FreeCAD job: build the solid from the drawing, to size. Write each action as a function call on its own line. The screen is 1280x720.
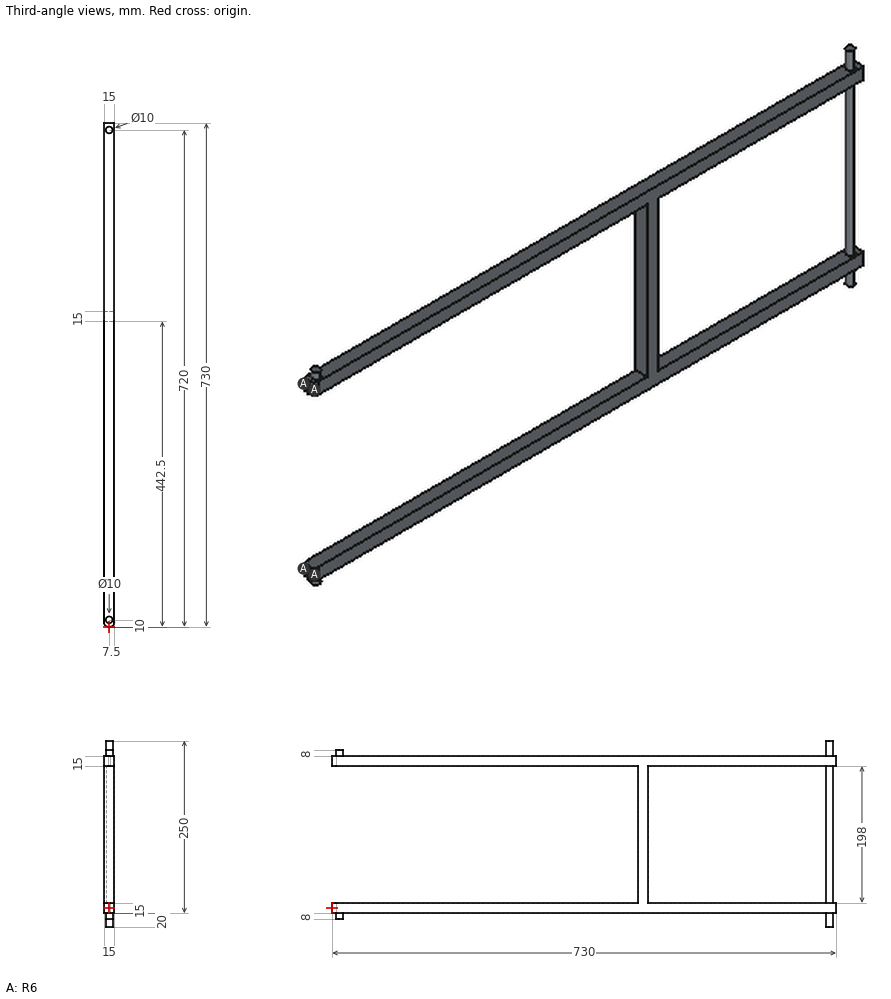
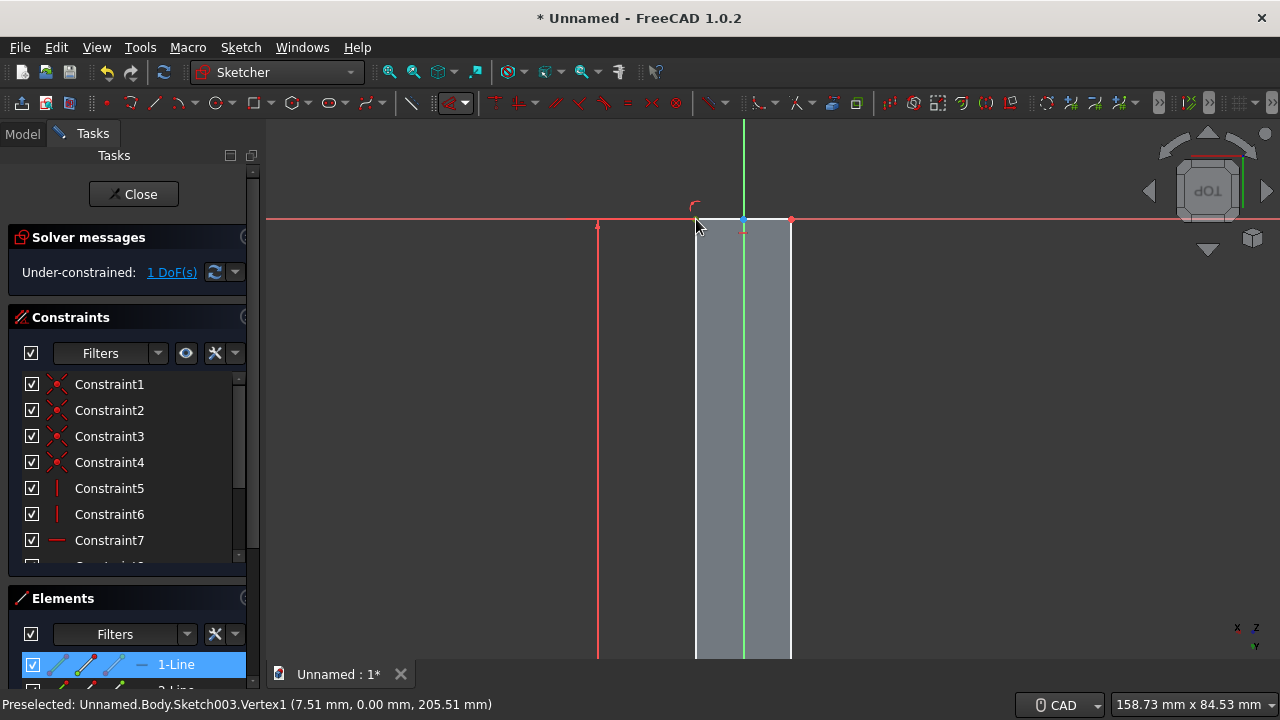
key(l)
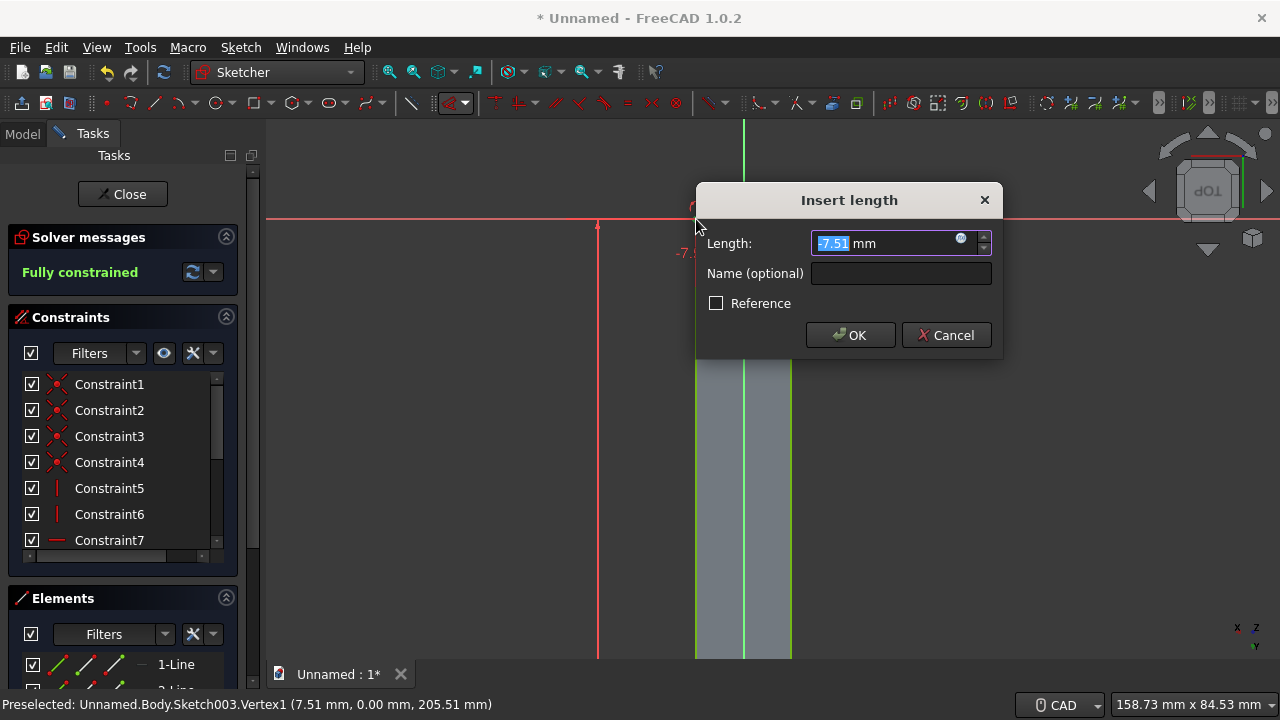
text(-7.5)
key(Return)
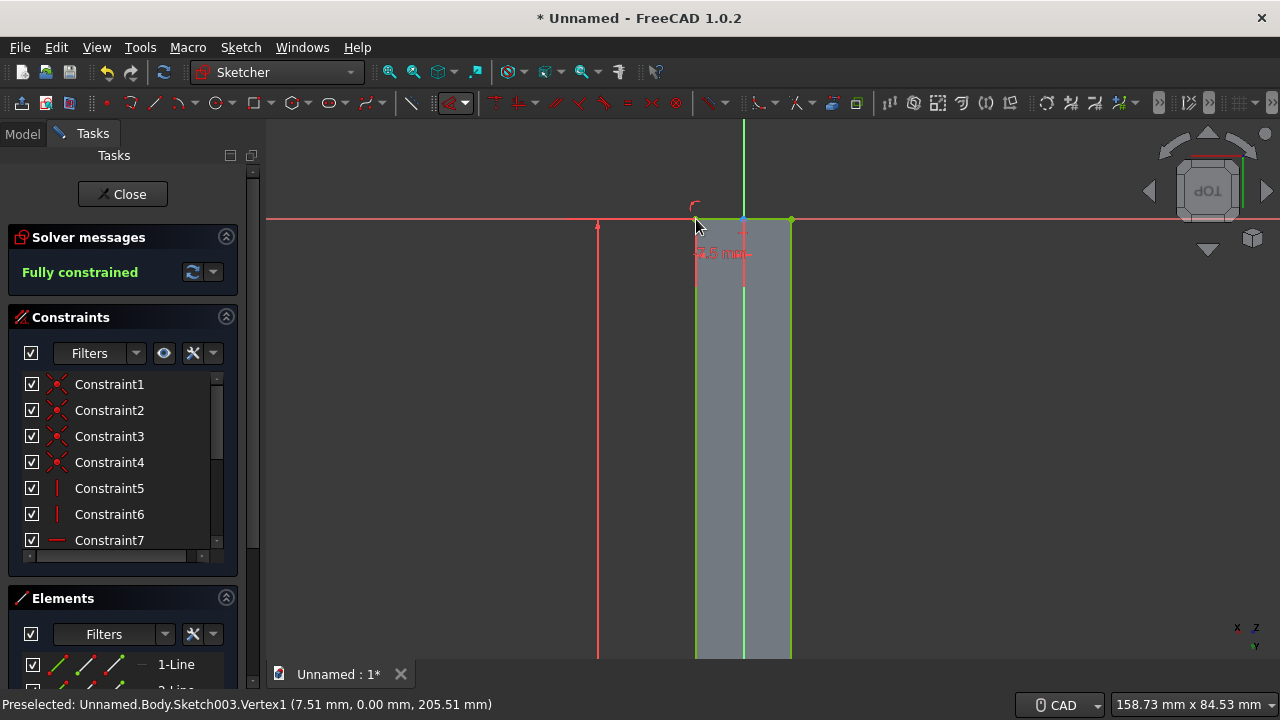
click(123, 194)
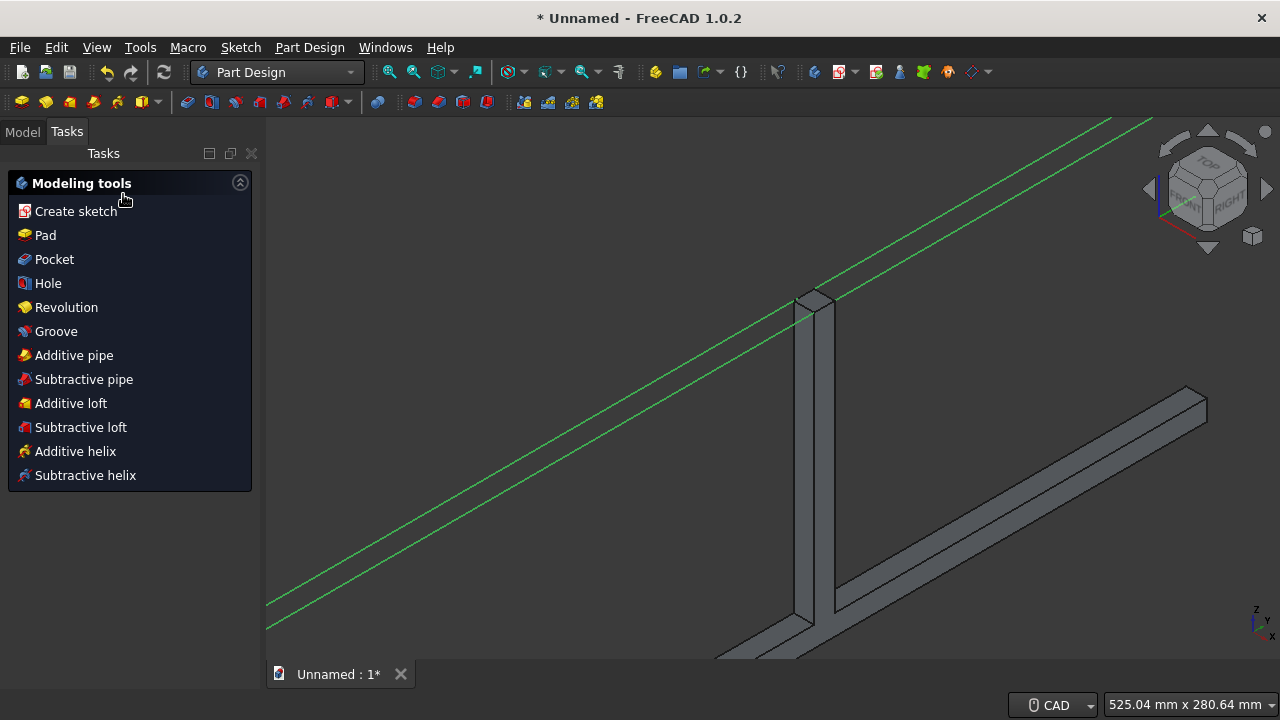
click(22, 102)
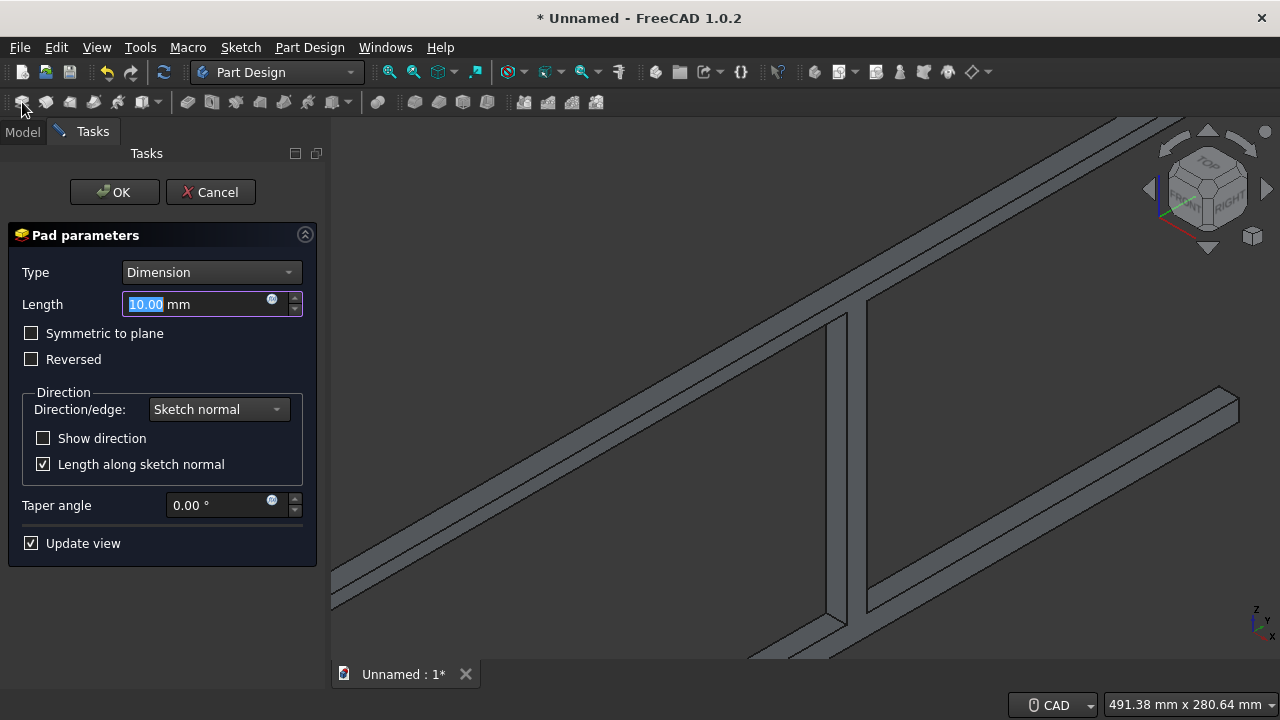
text(15)
key(Tab)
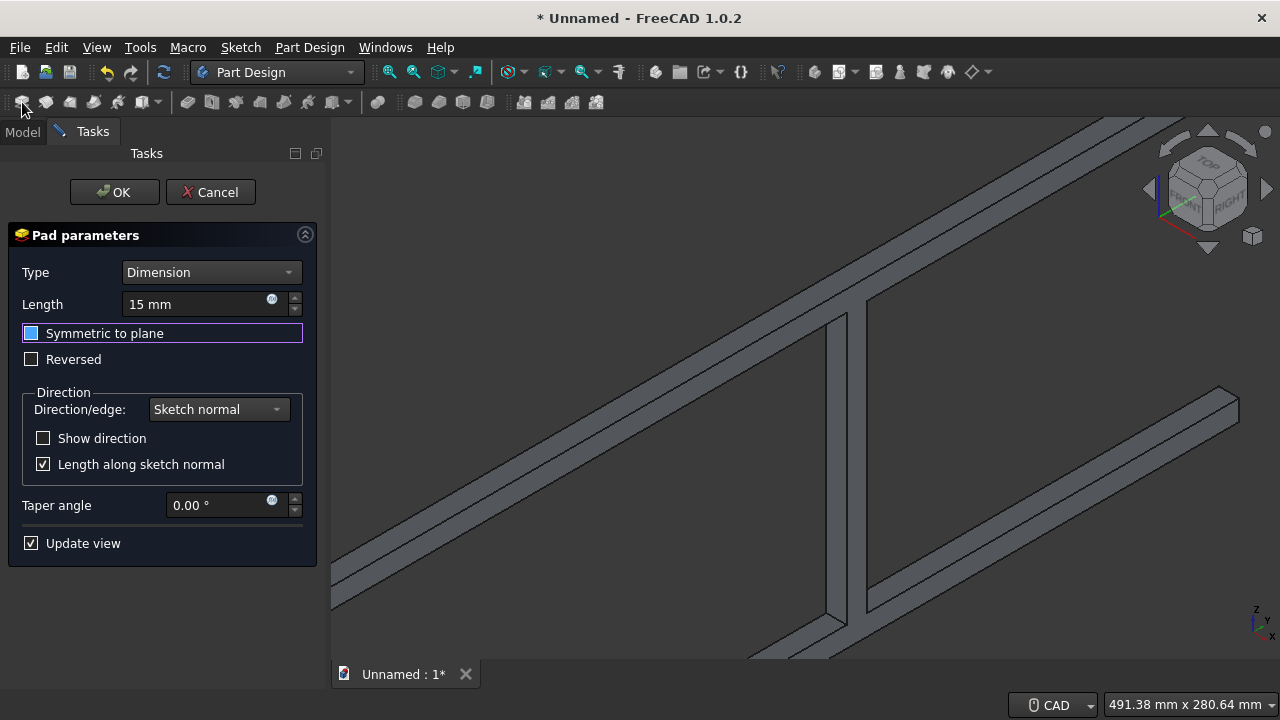
click(115, 192)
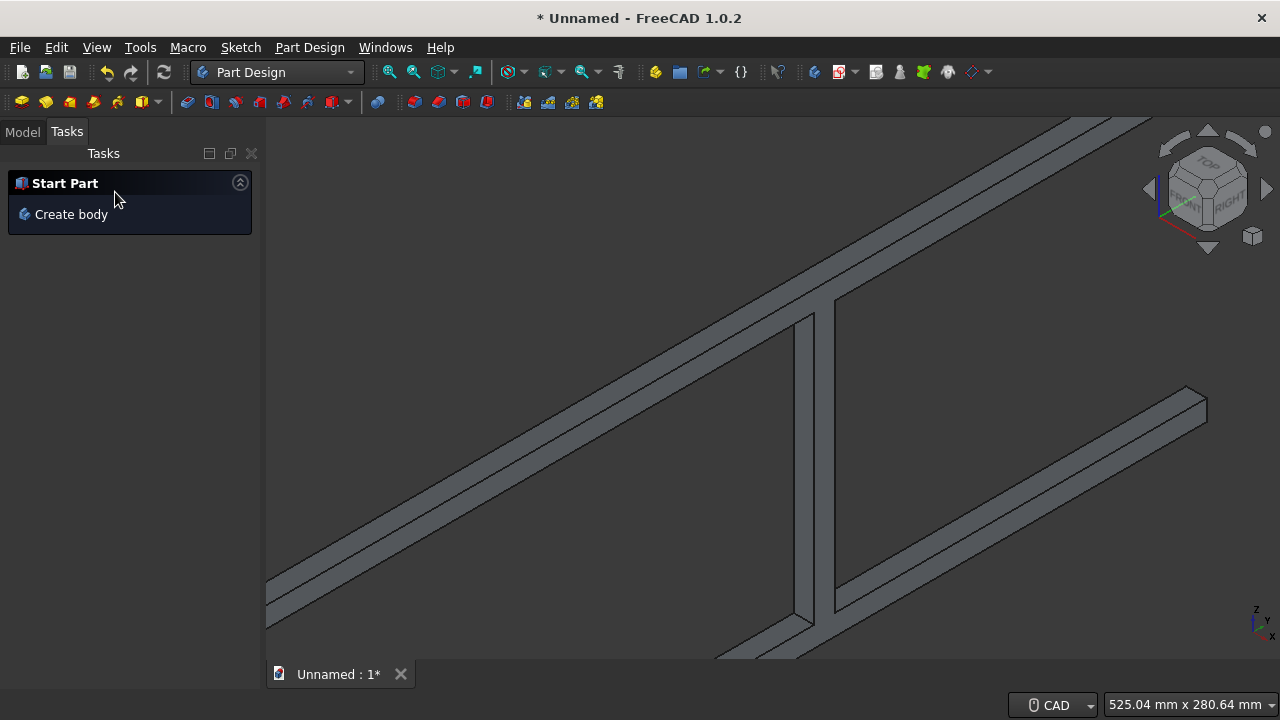
click(390, 72)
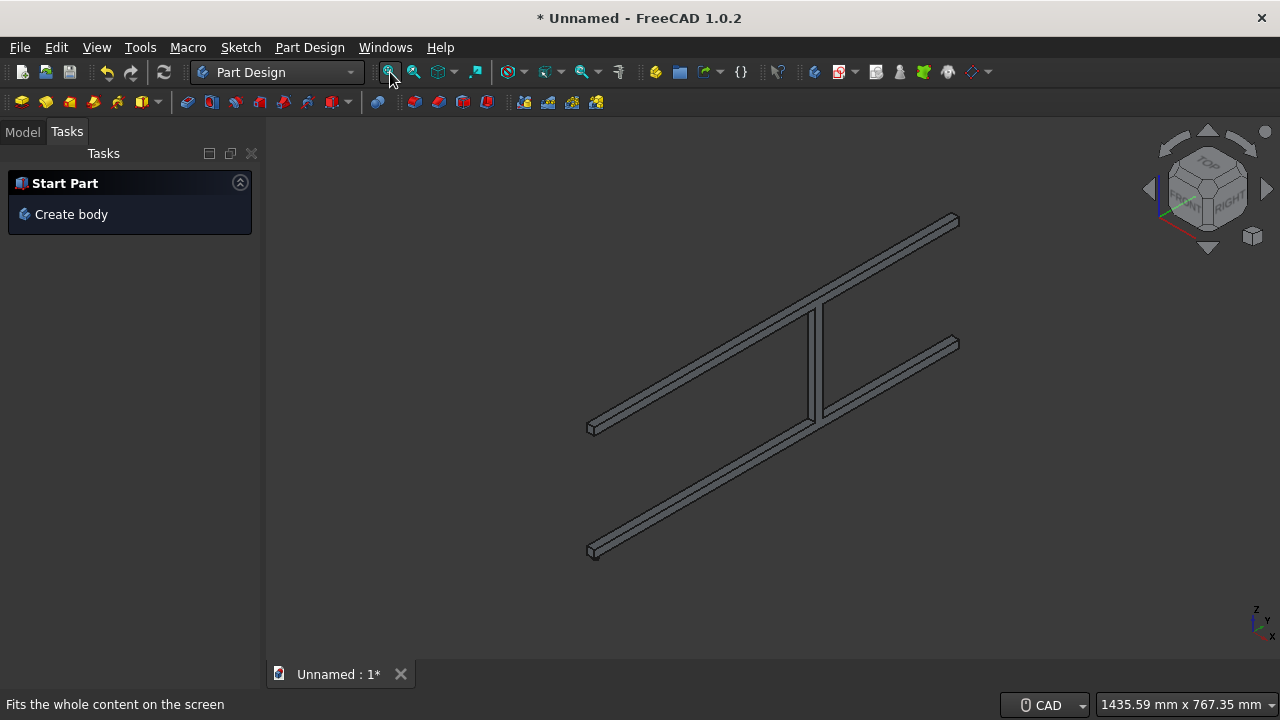
click(23, 131)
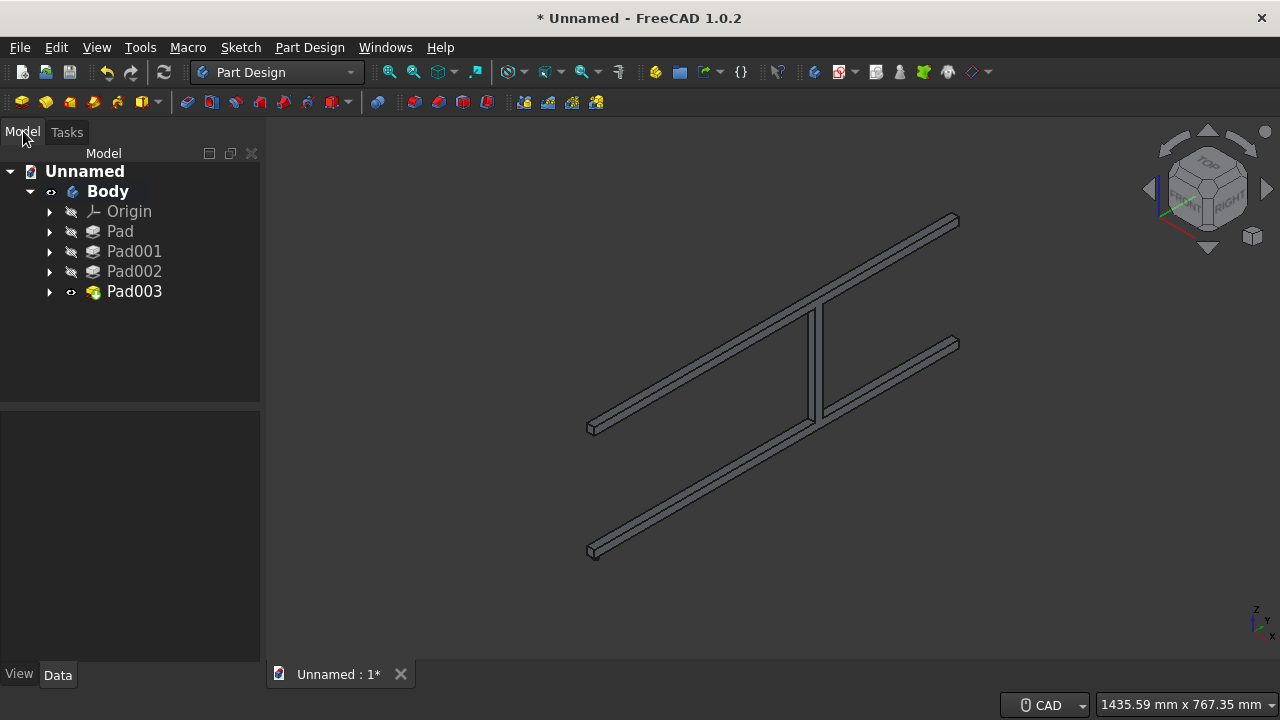
click(50, 212)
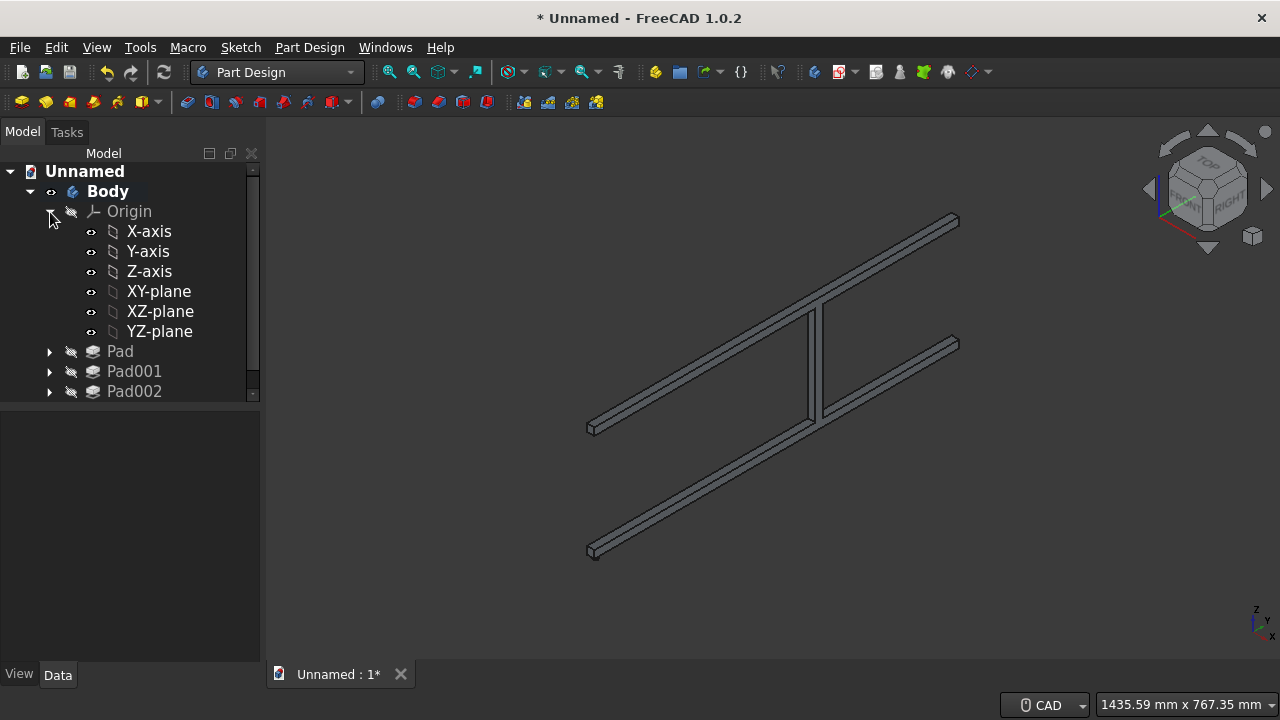
click(136, 292)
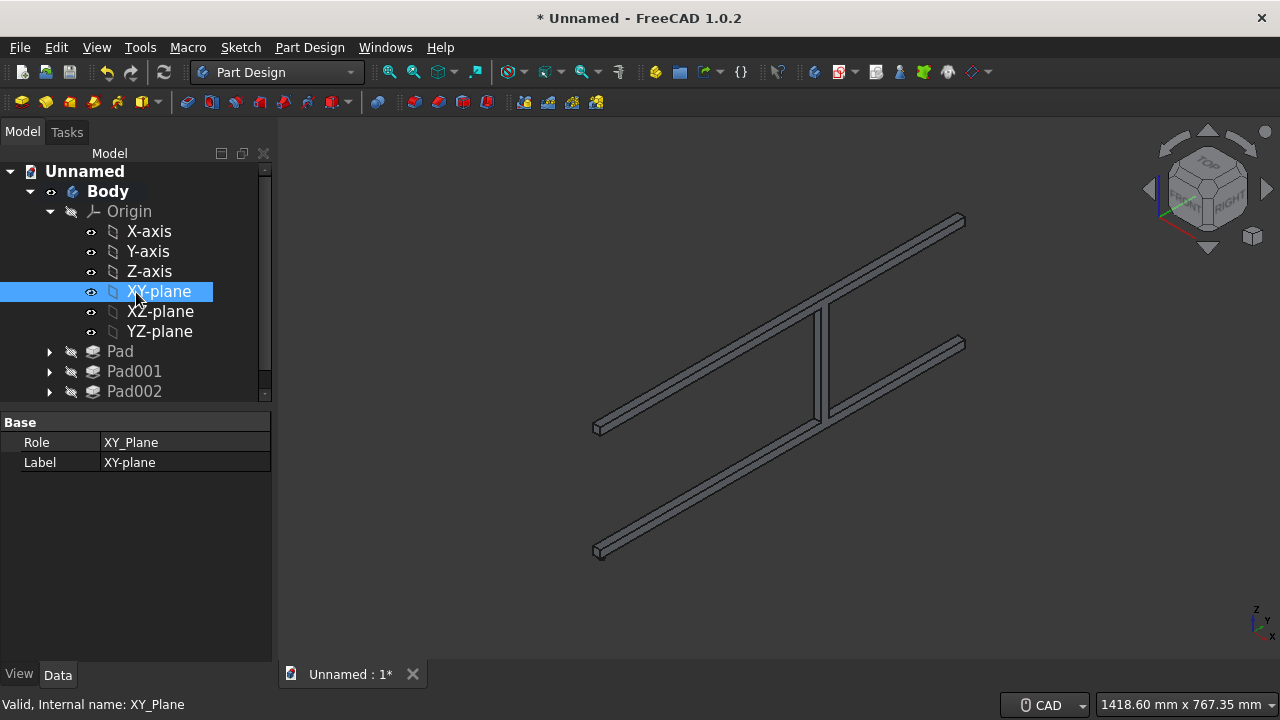
click(972, 72)